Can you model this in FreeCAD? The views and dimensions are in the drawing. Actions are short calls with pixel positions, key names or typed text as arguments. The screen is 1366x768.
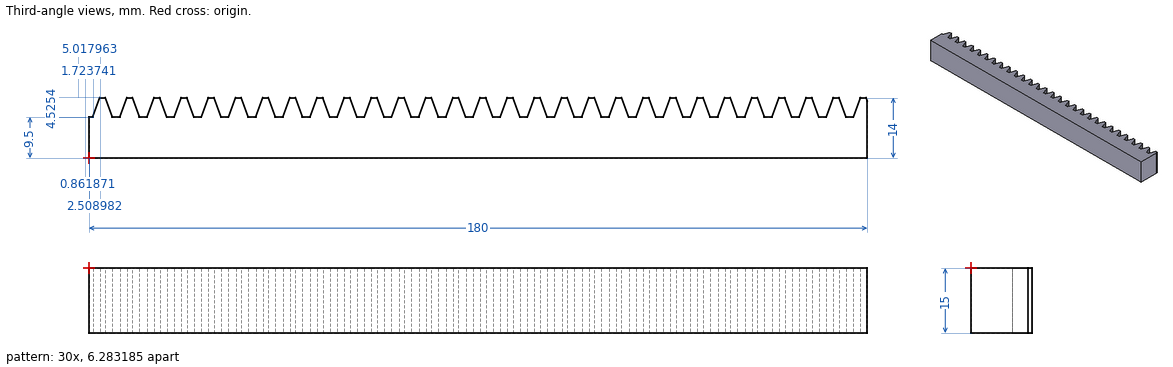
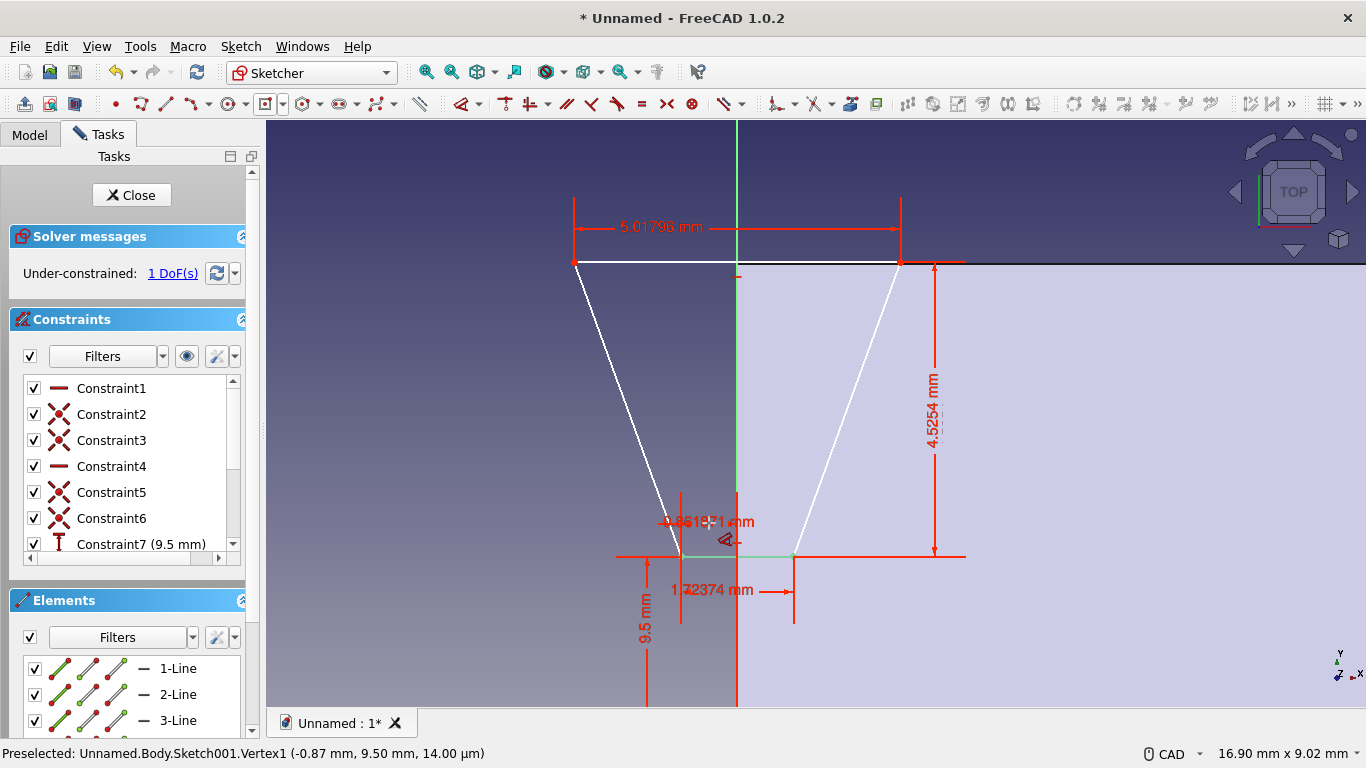
click(901, 262)
click(819, 228)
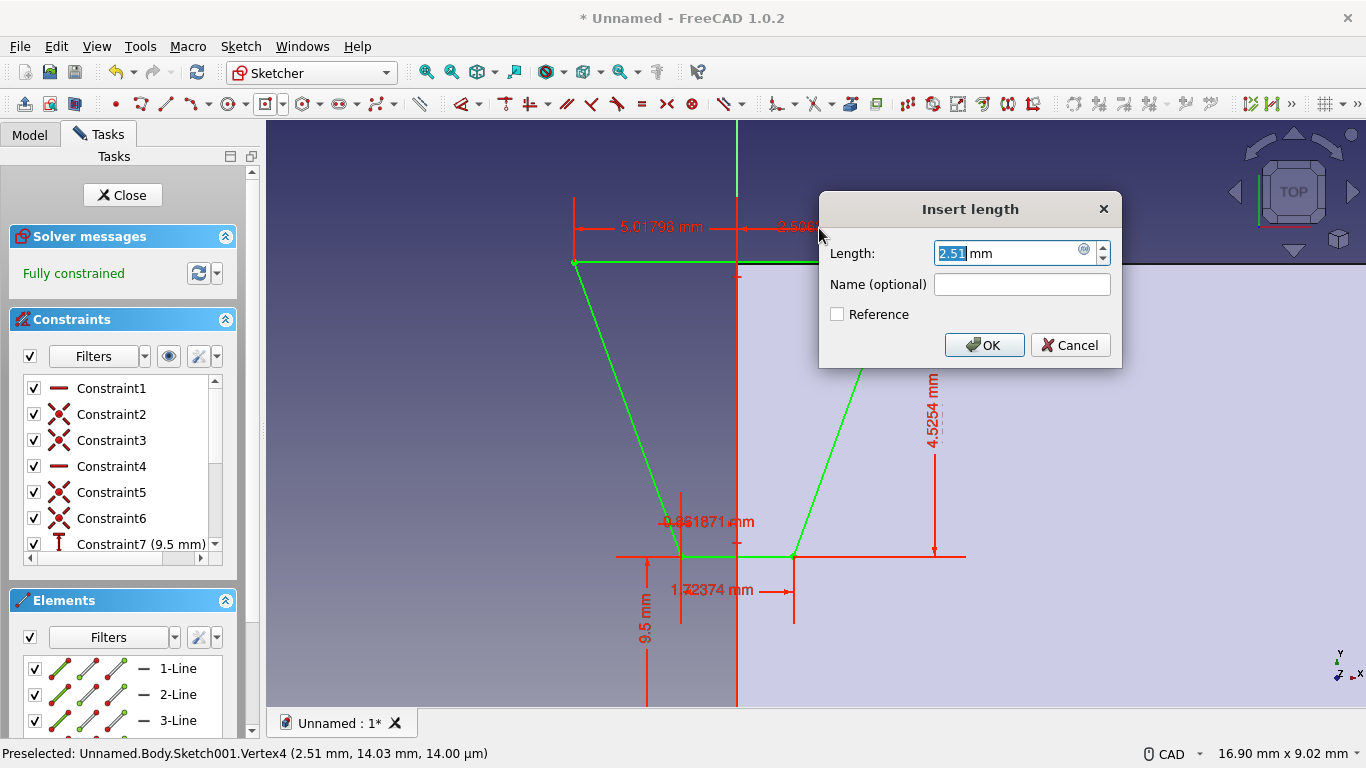
text(2.508982)
key(Return)
key(Escape)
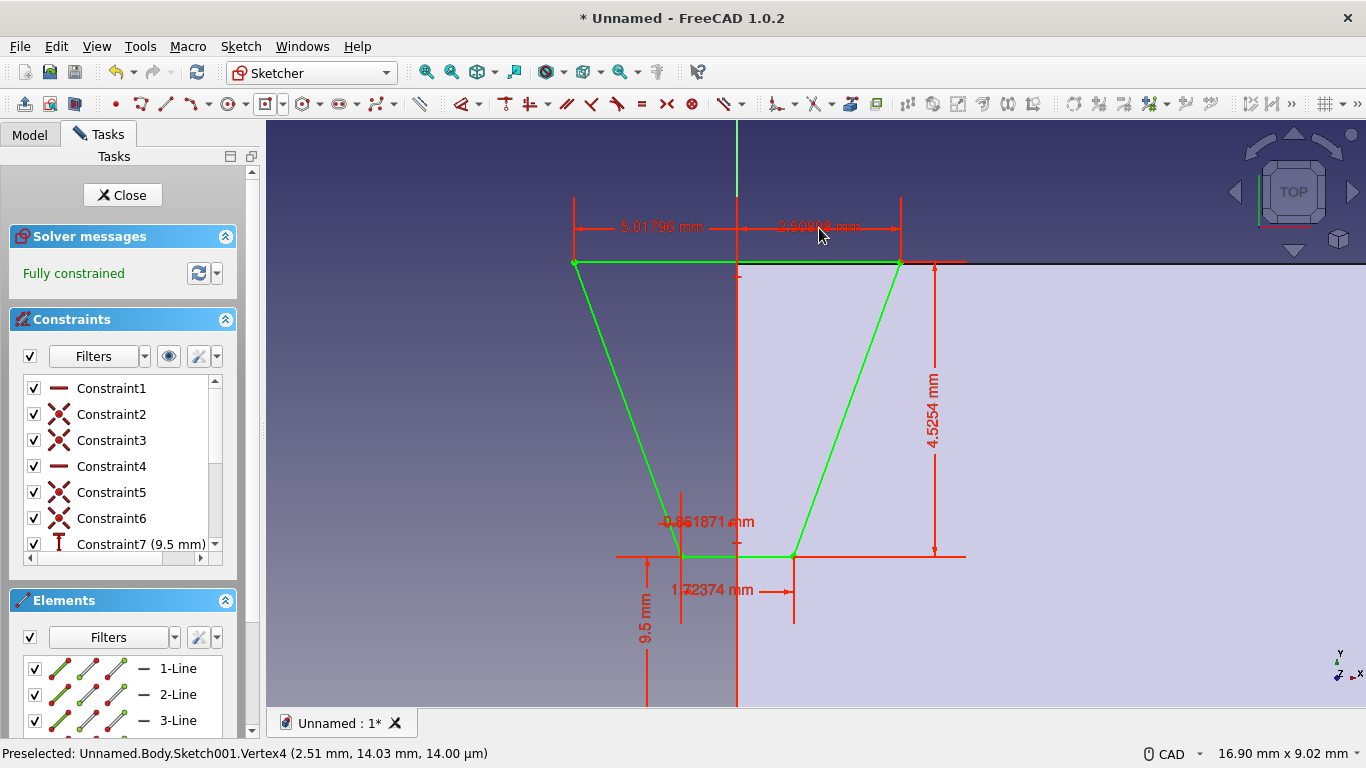
click(123, 195)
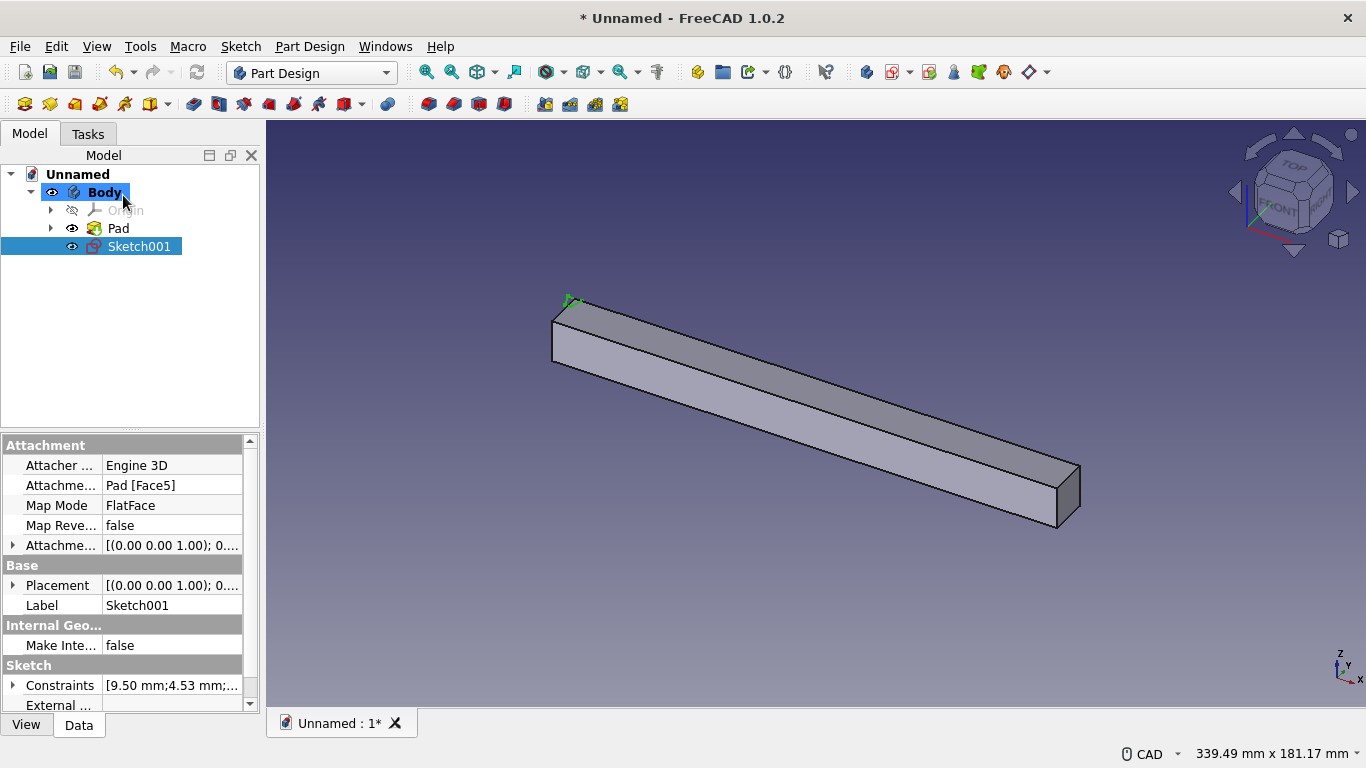
click(194, 104)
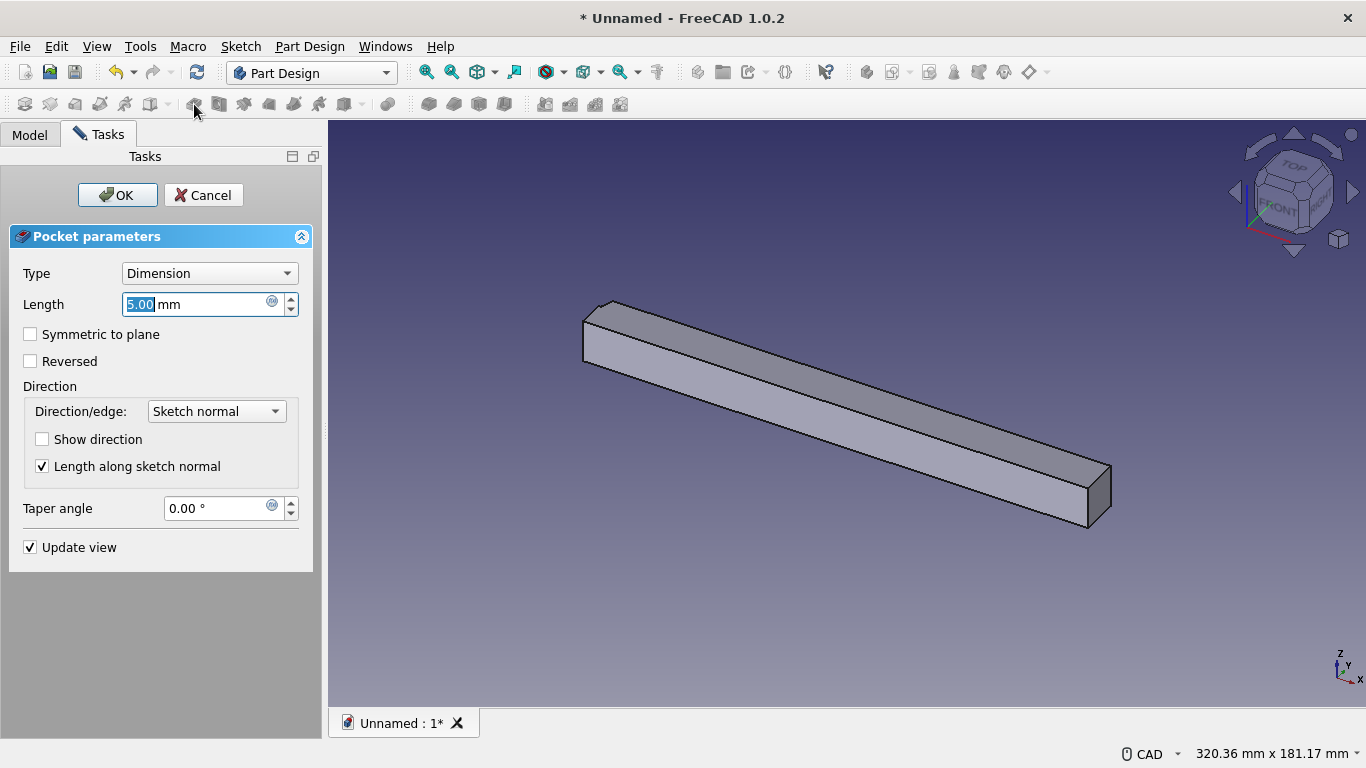
click(210, 274)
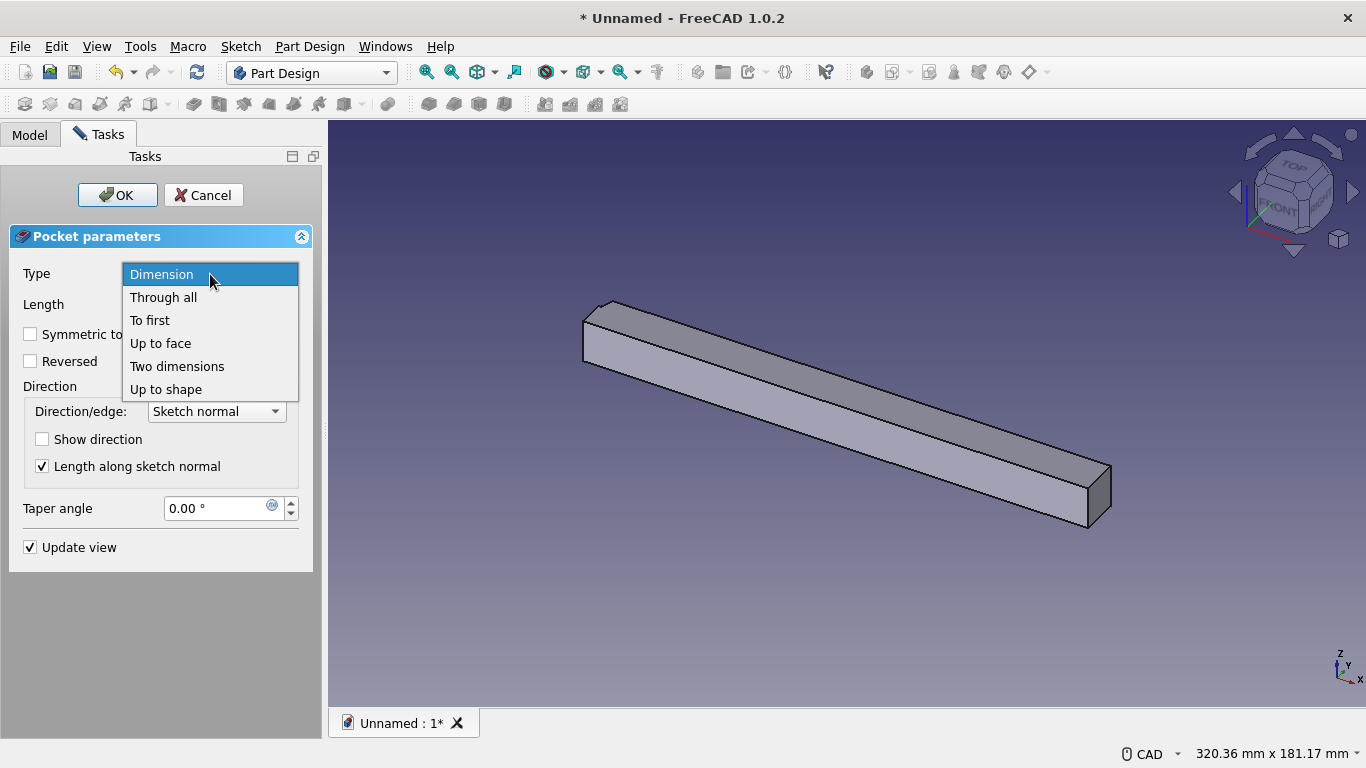
click(208, 298)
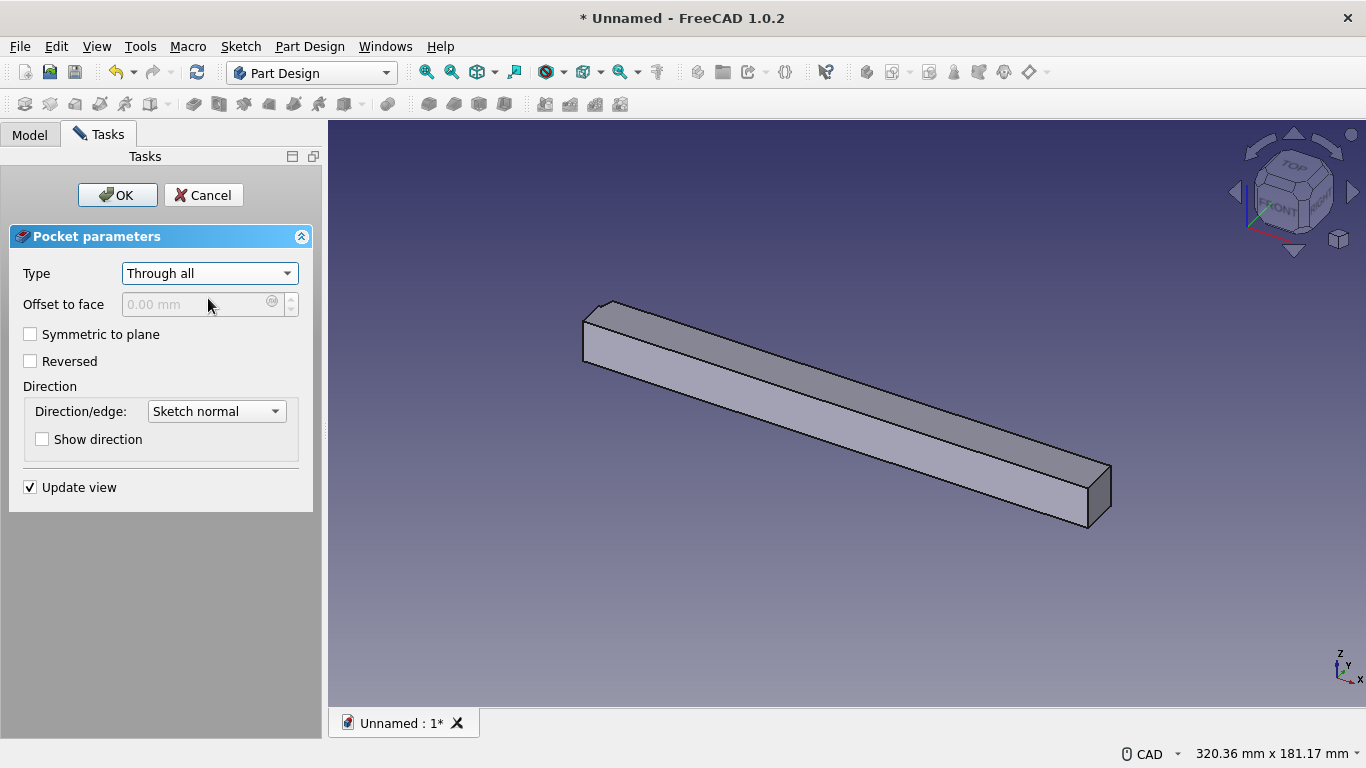
click(118, 195)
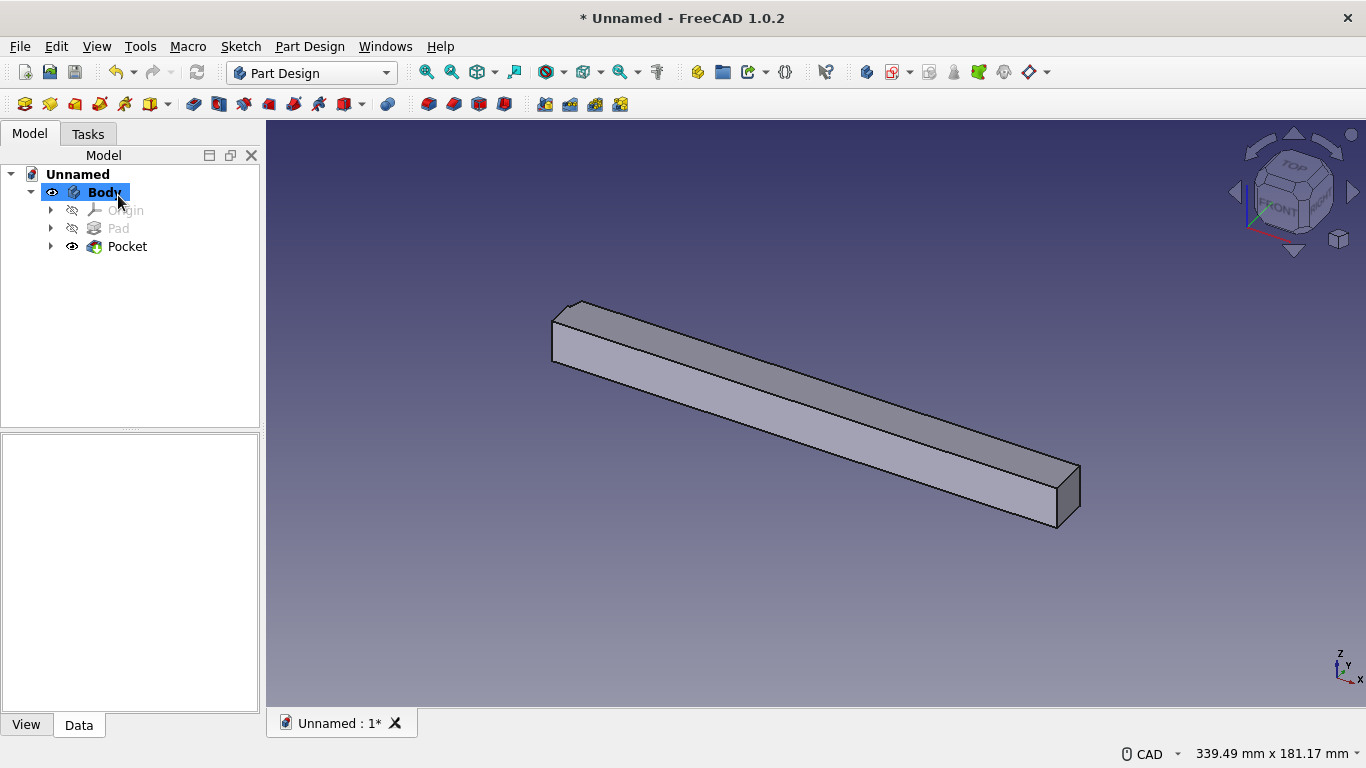
click(117, 246)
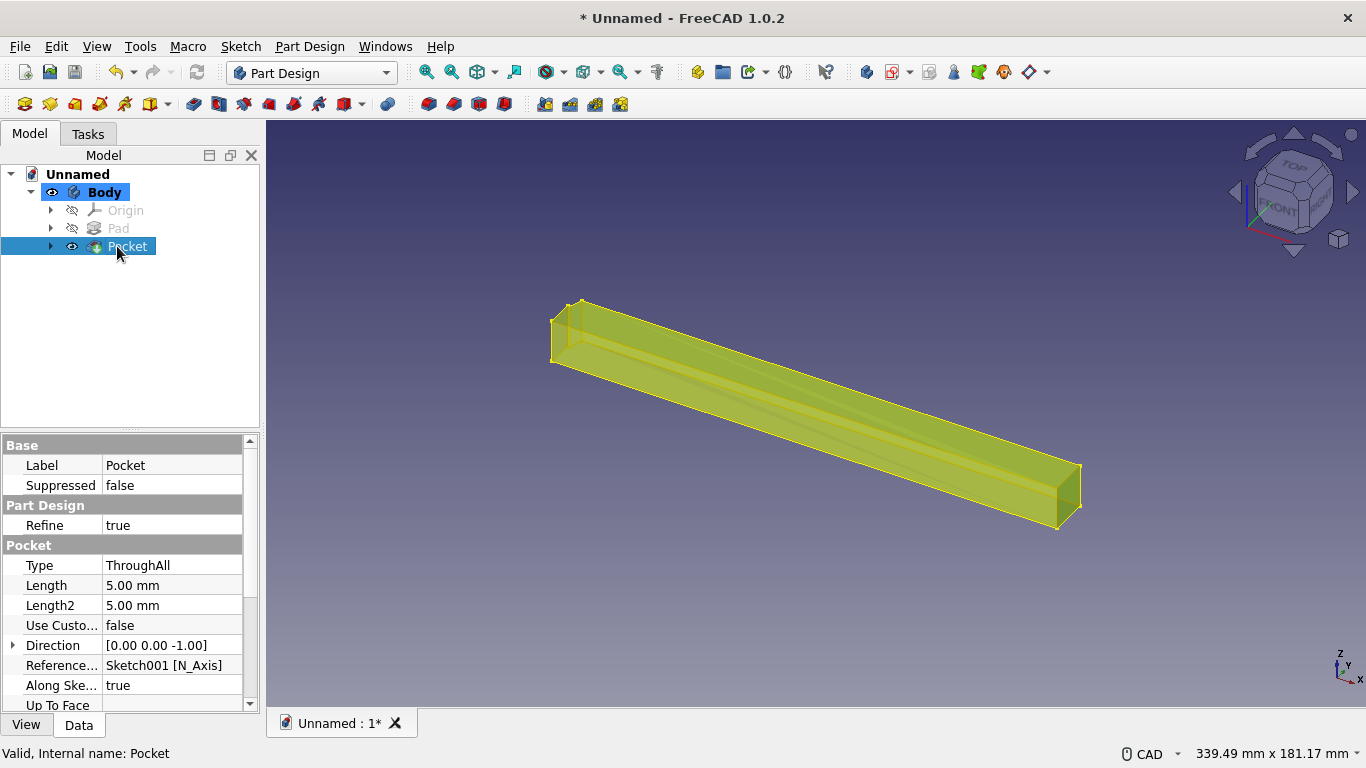
click(570, 104)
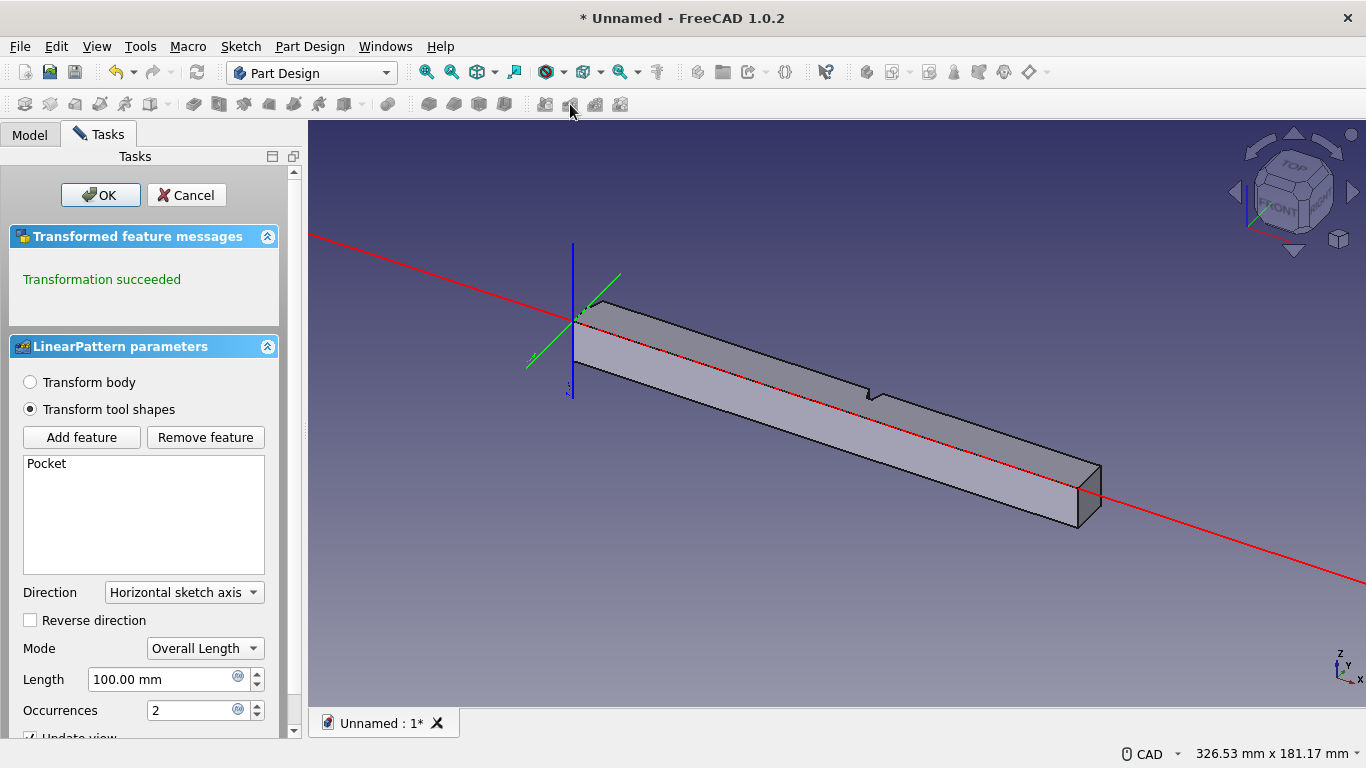
click(185, 592)